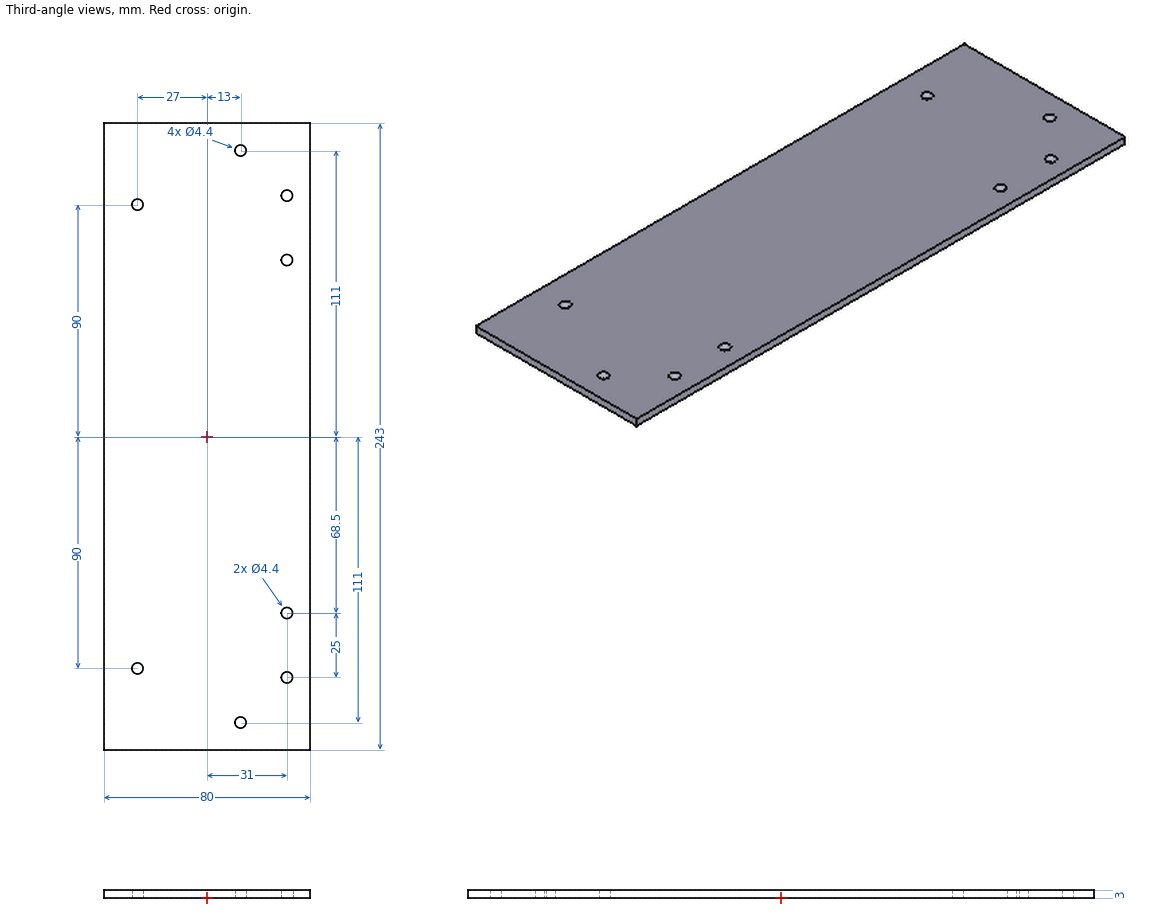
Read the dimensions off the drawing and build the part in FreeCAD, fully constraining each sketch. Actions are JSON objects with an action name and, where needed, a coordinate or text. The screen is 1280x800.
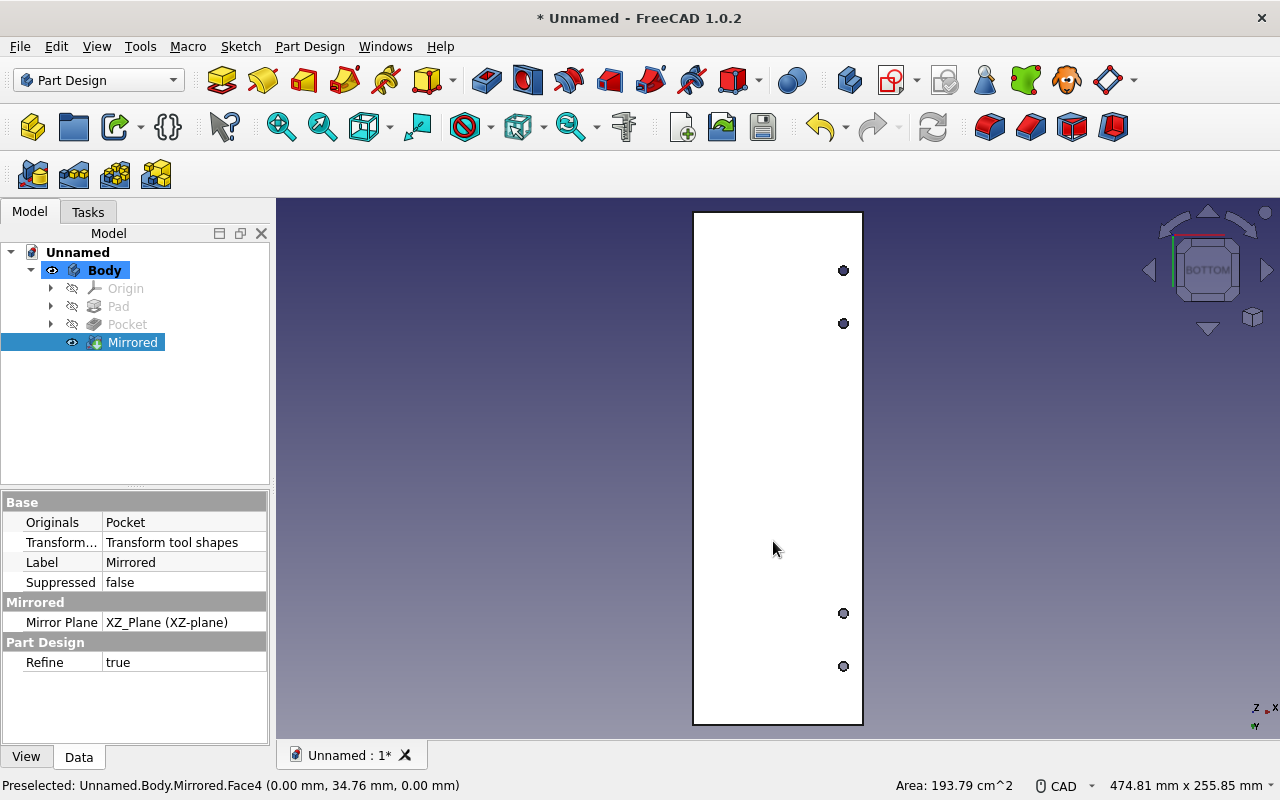
{"action": "left_click", "coordinate": [890, 80]}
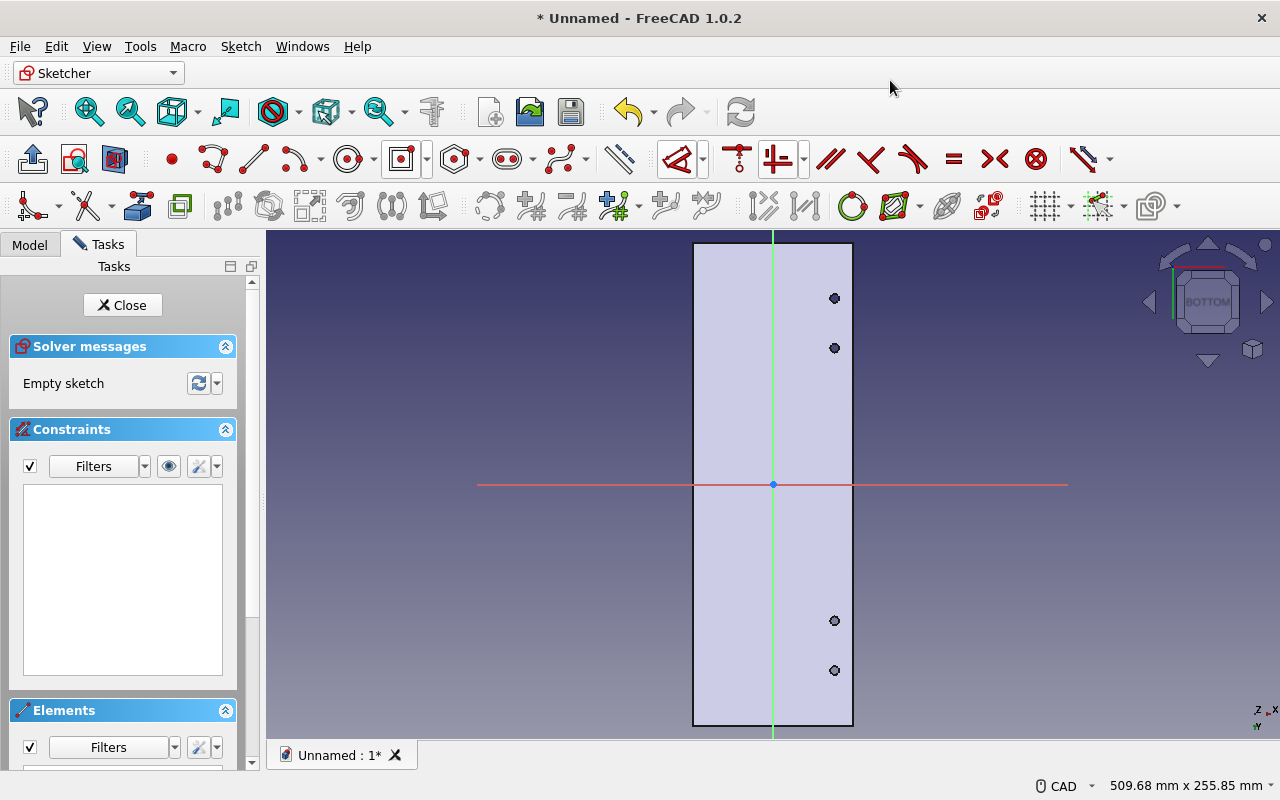
{"action": "scroll", "coordinate": [594, 484], "scroll_direction": "down", "scroll_amount": 2}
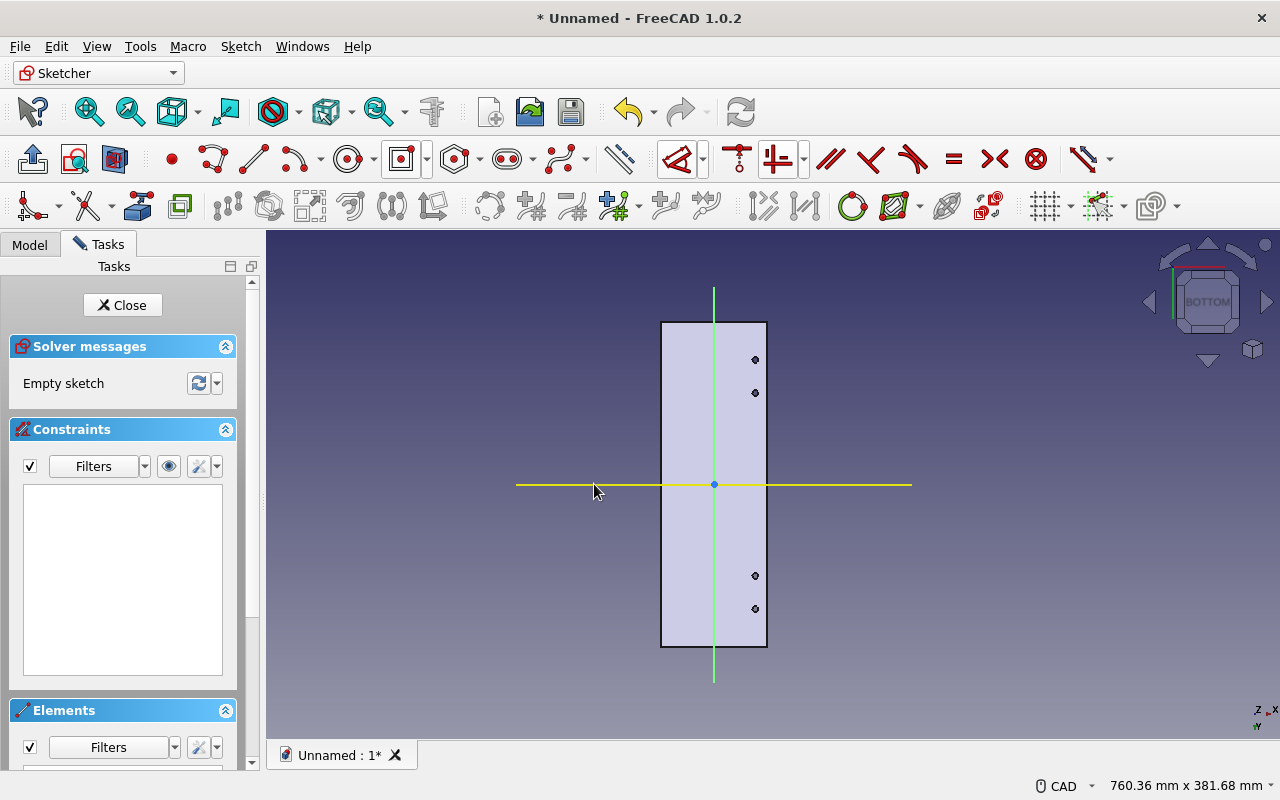
{"action": "left_click", "coordinate": [348, 160]}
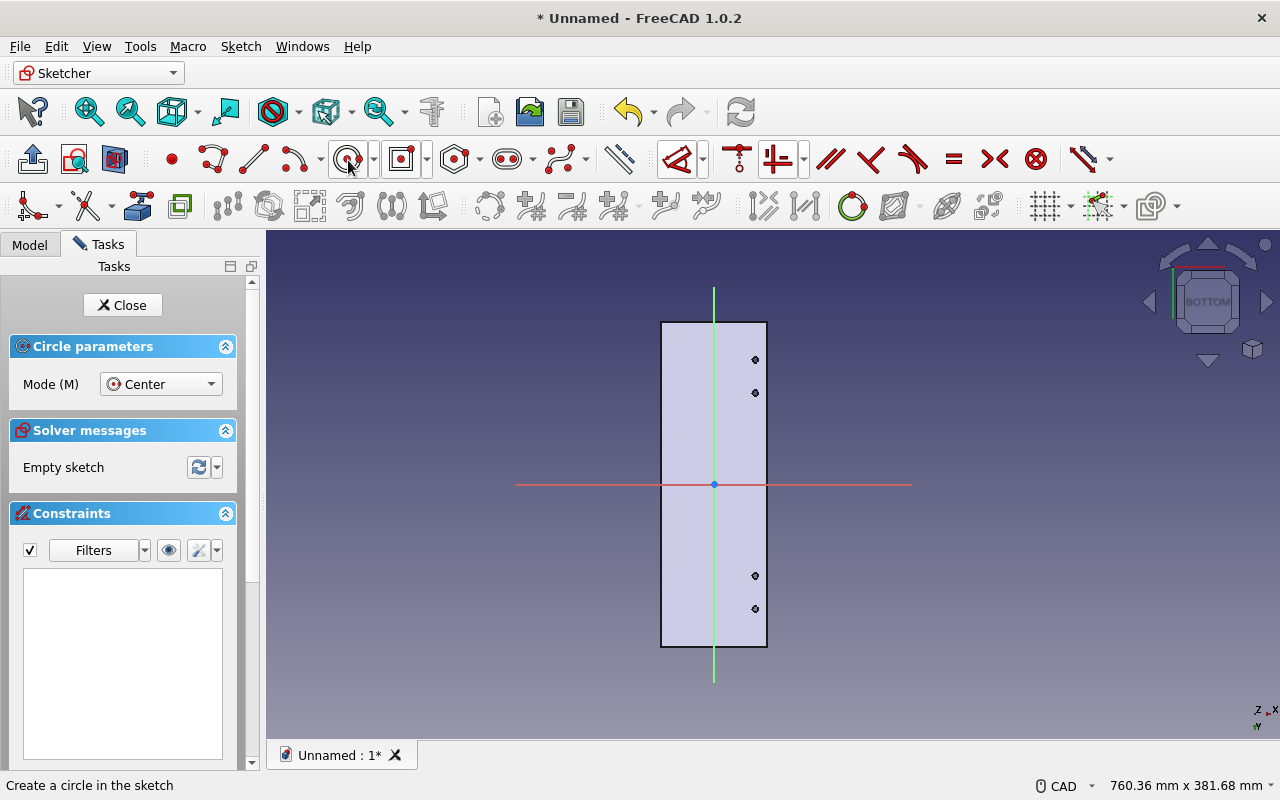
{"action": "scroll", "coordinate": [731, 633], "scroll_direction": "up", "scroll_amount": 11}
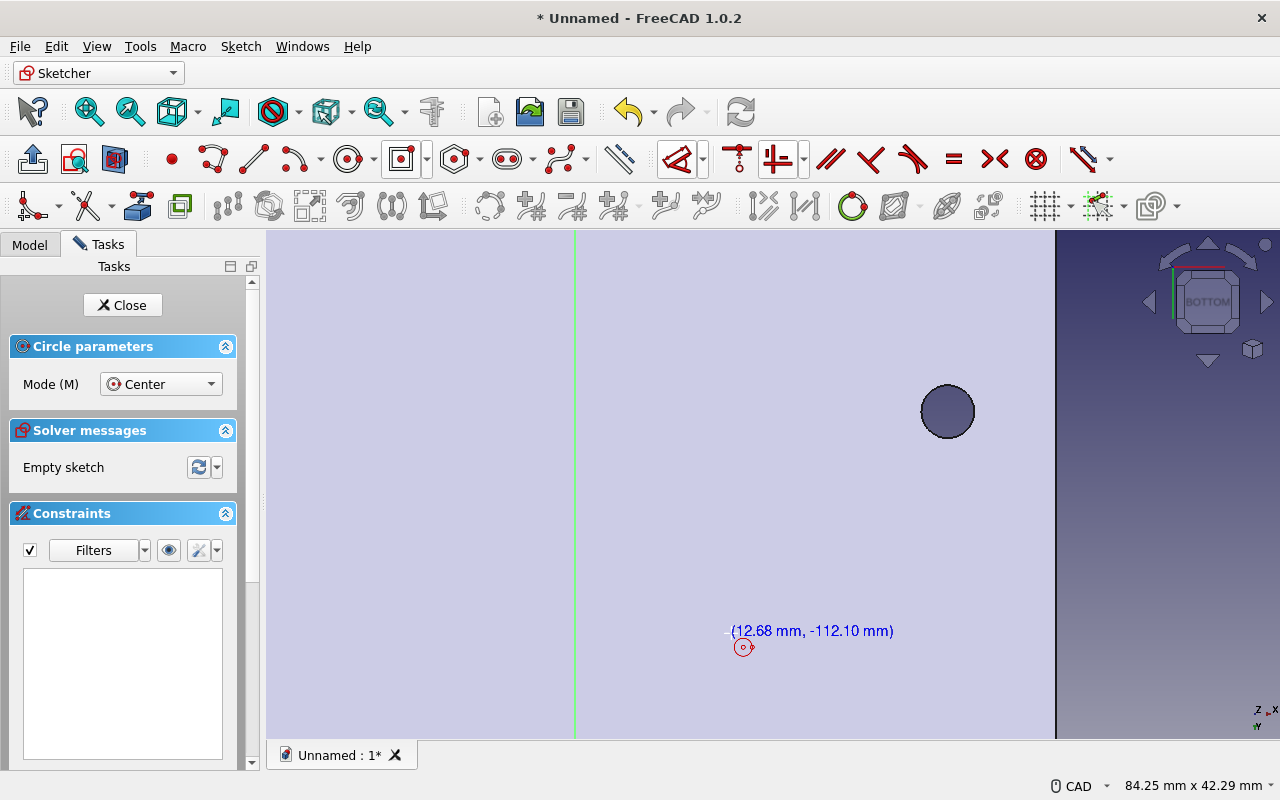
{"action": "scroll", "coordinate": [731, 634], "scroll_direction": "down", "scroll_amount": 11}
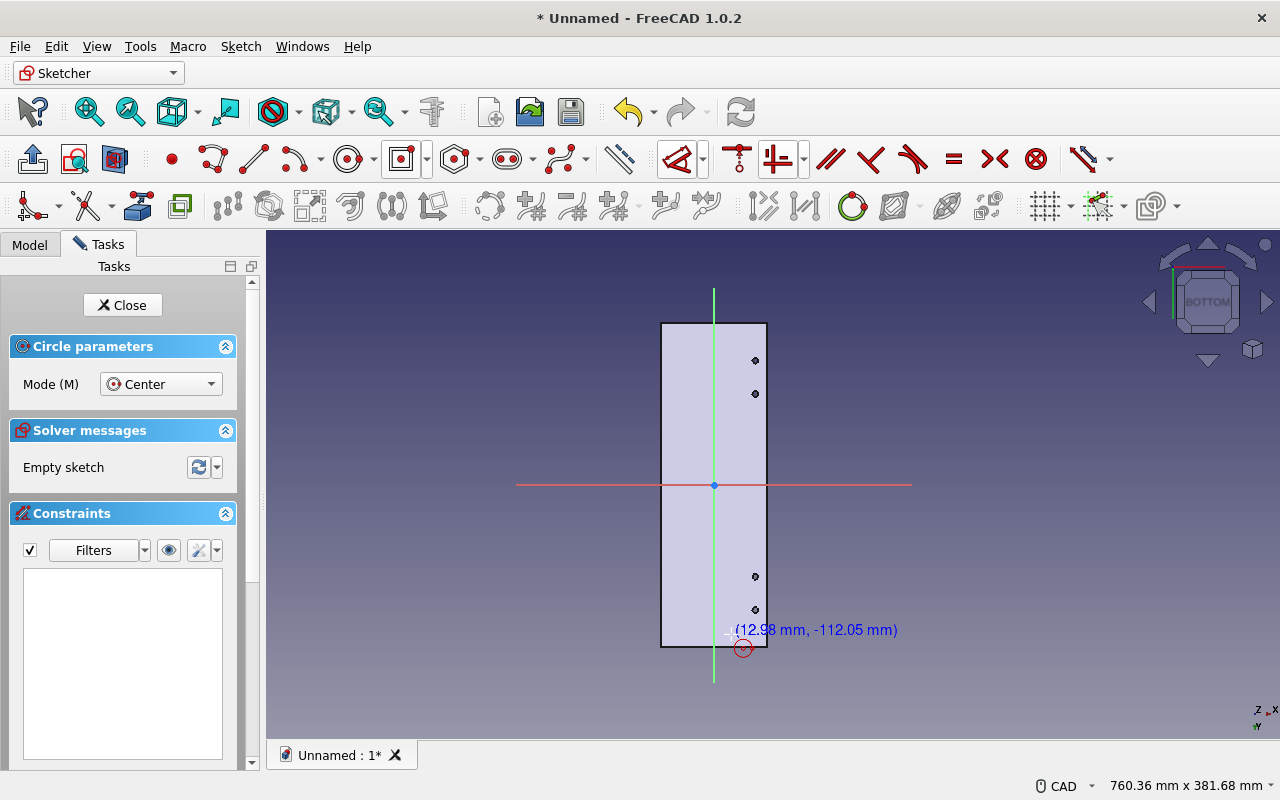
{"action": "left_click", "coordinate": [731, 633]}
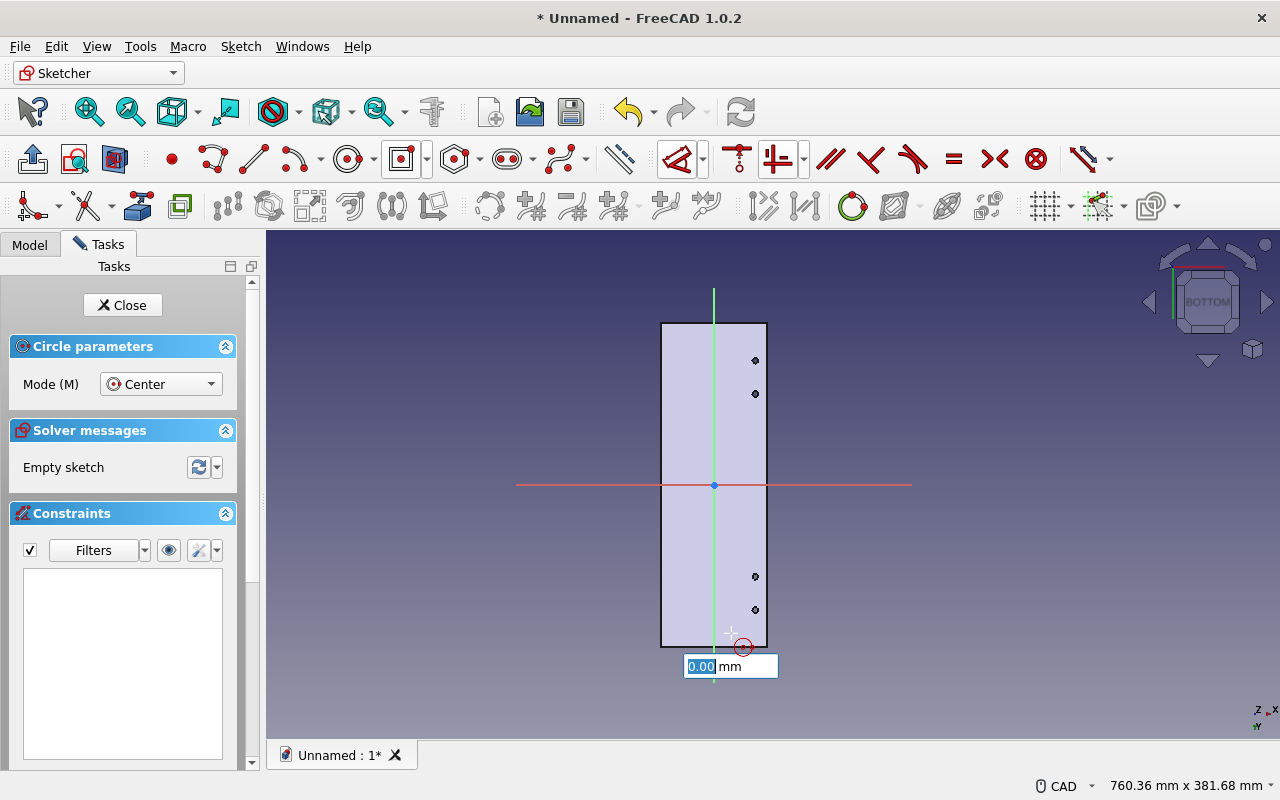
{"action": "scroll", "coordinate": [734, 631], "scroll_direction": "up", "scroll_amount": 9}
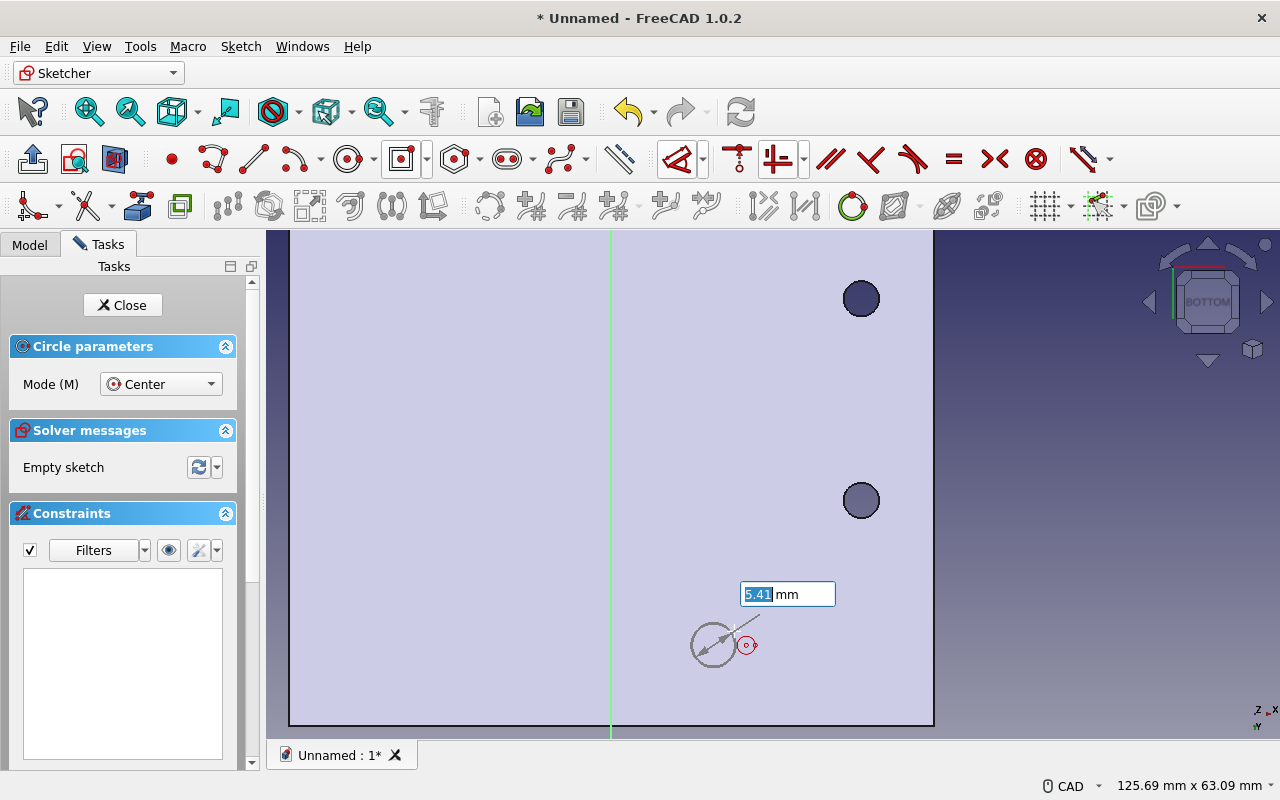
{"action": "left_click", "coordinate": [729, 629]}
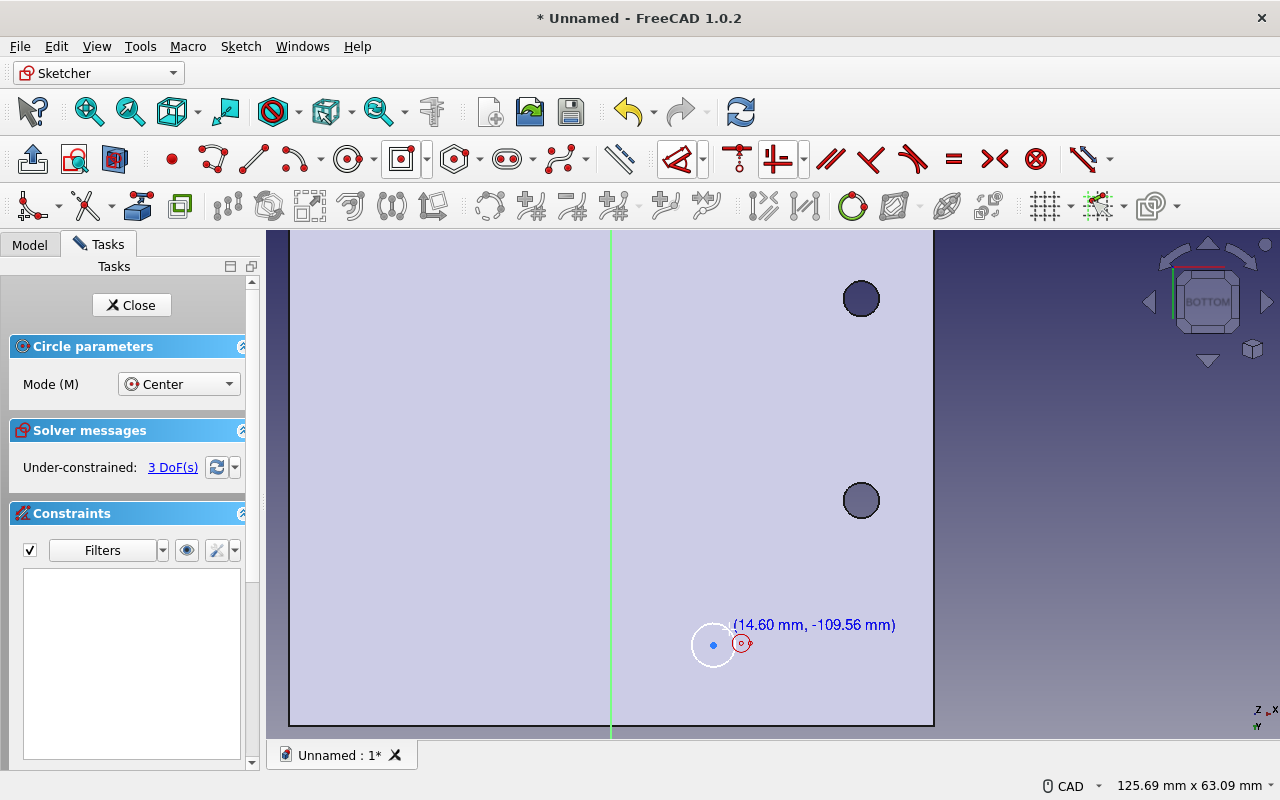
{"action": "scroll", "coordinate": [734, 631], "scroll_direction": "down", "scroll_amount": 9}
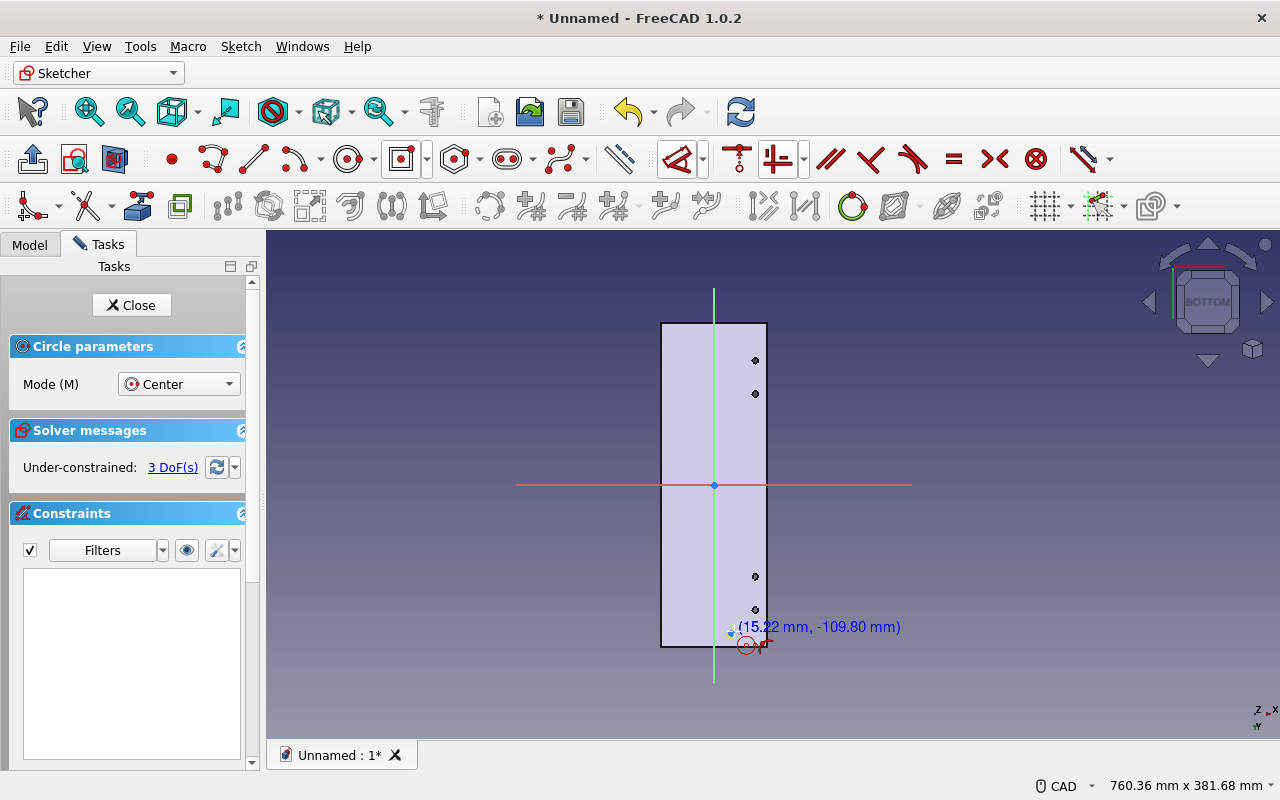
{"action": "scroll", "coordinate": [731, 337], "scroll_direction": "up", "scroll_amount": 11}